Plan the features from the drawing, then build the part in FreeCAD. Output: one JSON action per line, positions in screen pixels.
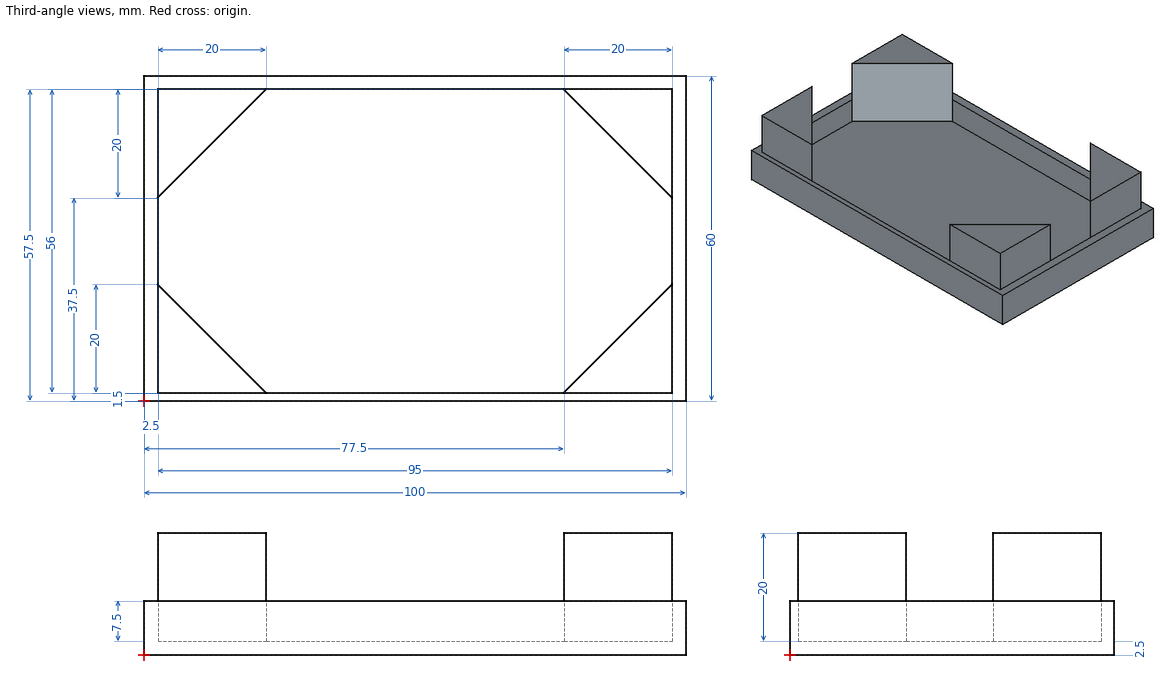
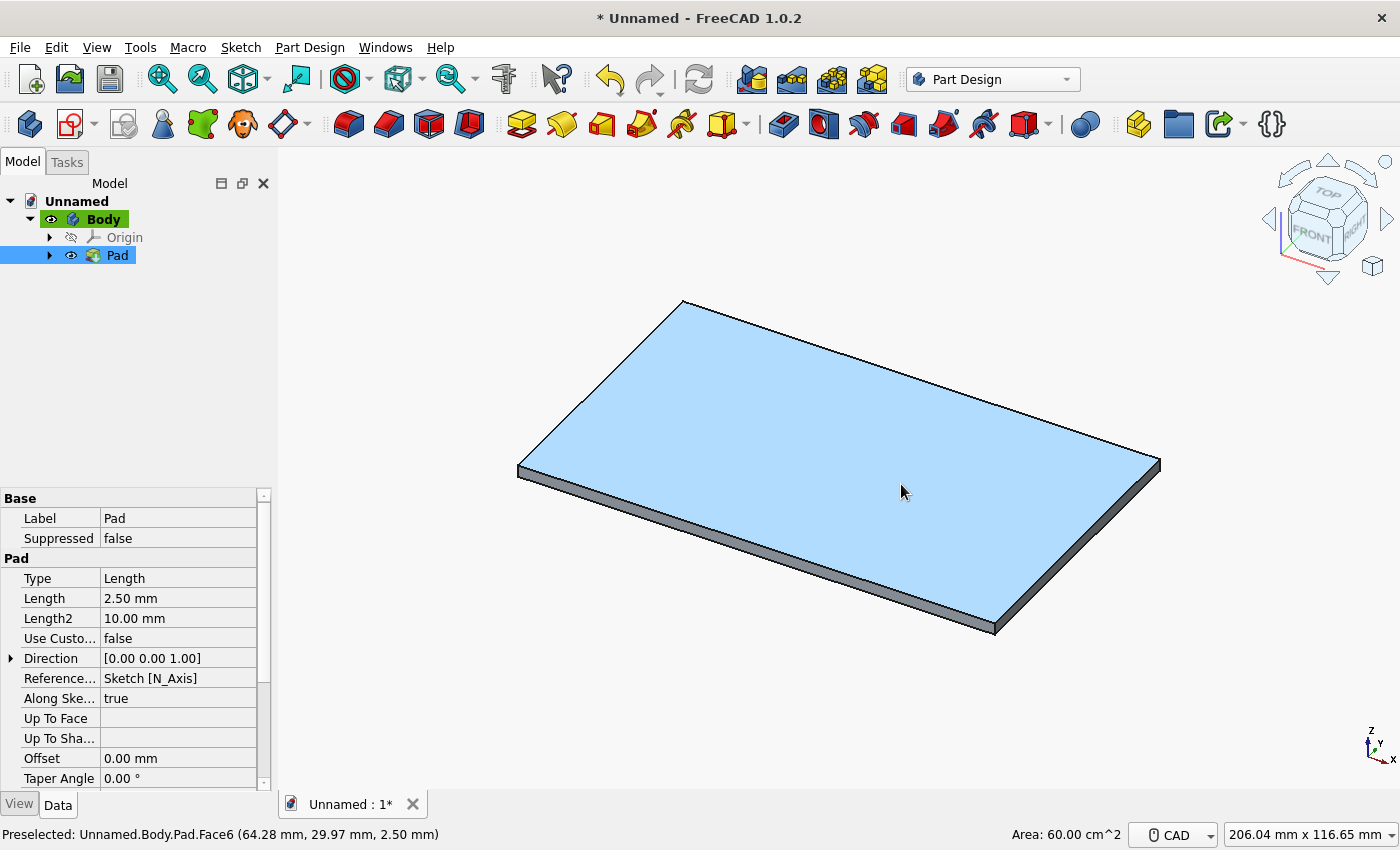
{"action": "left_click", "coordinate": [70, 124]}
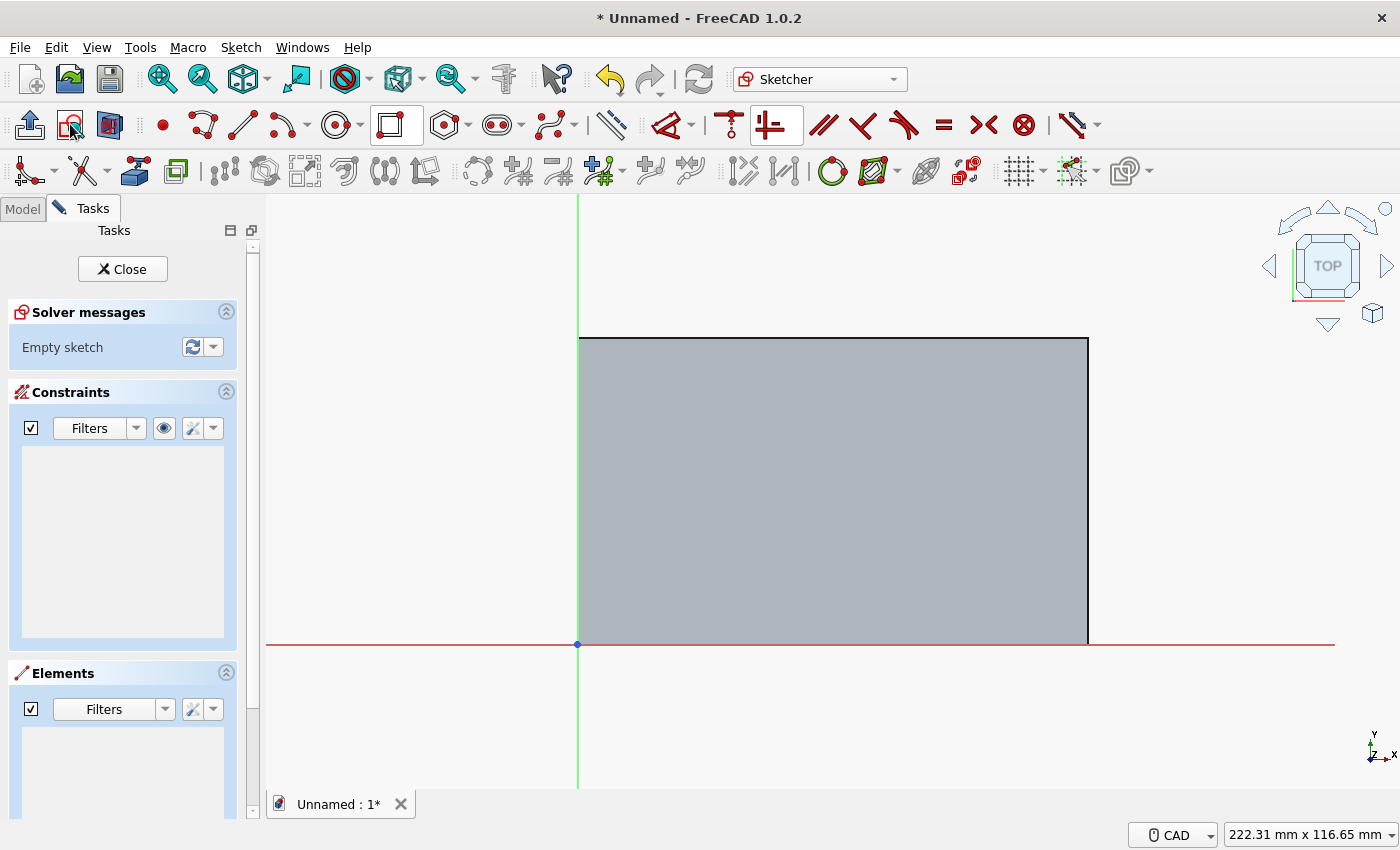
{"action": "left_click", "coordinate": [390, 126]}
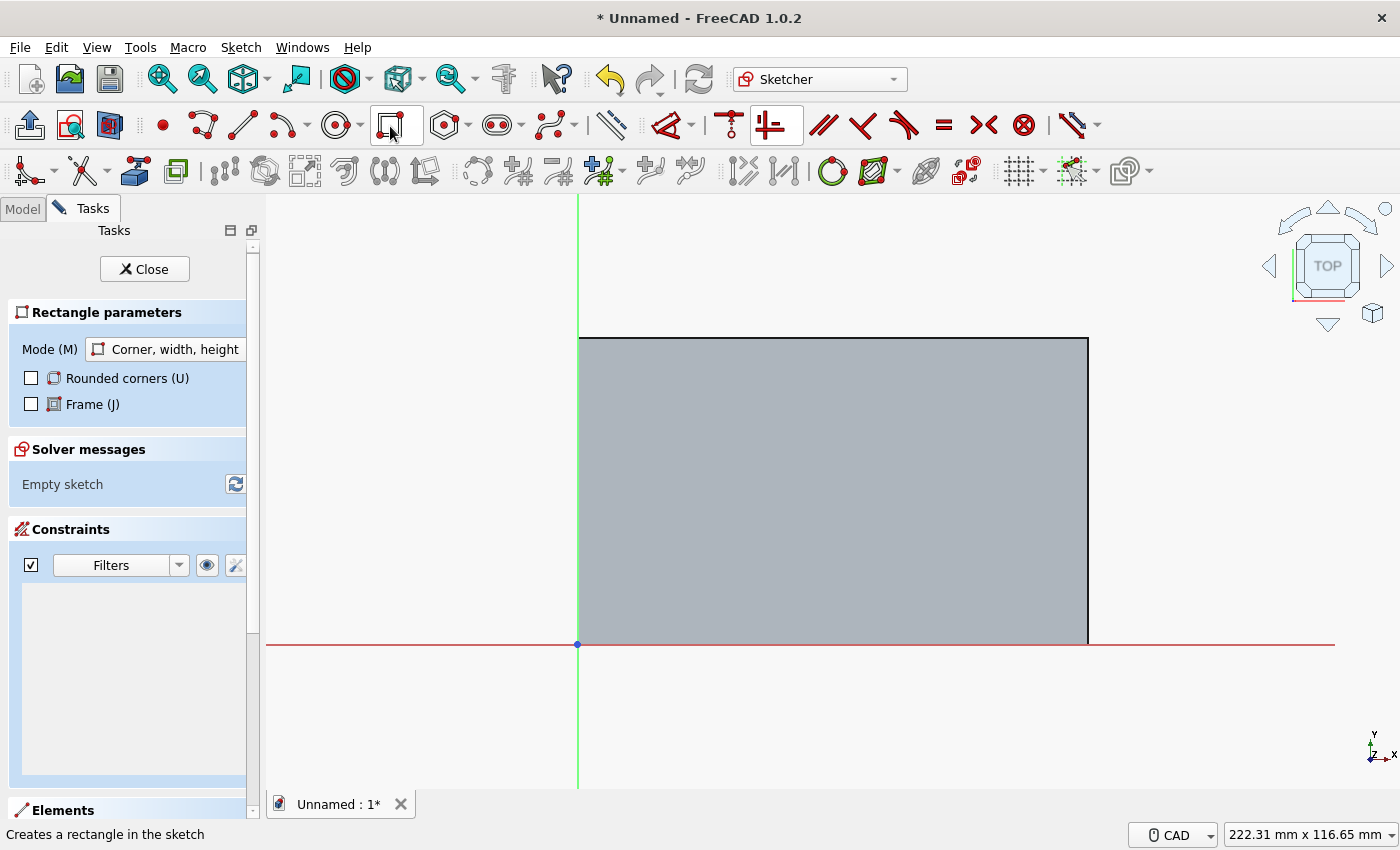
{"action": "left_click", "coordinate": [578, 645]}
{"action": "mouse_move", "coordinate": [1088, 338]}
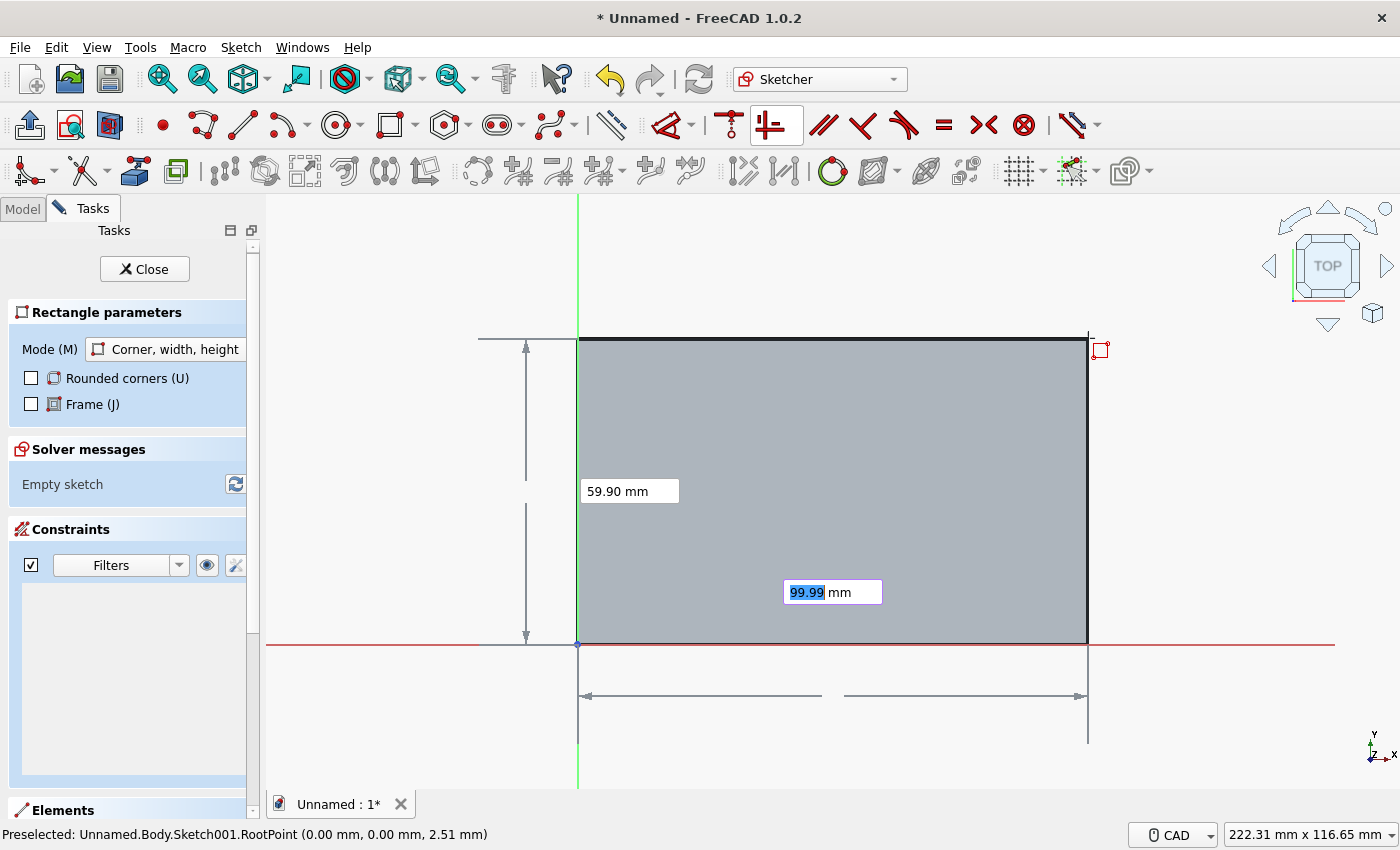
{"action": "type", "text": "100"}
{"action": "key", "text": "Tab"}
{"action": "type", "text": "60"}
{"action": "key", "text": "Return"}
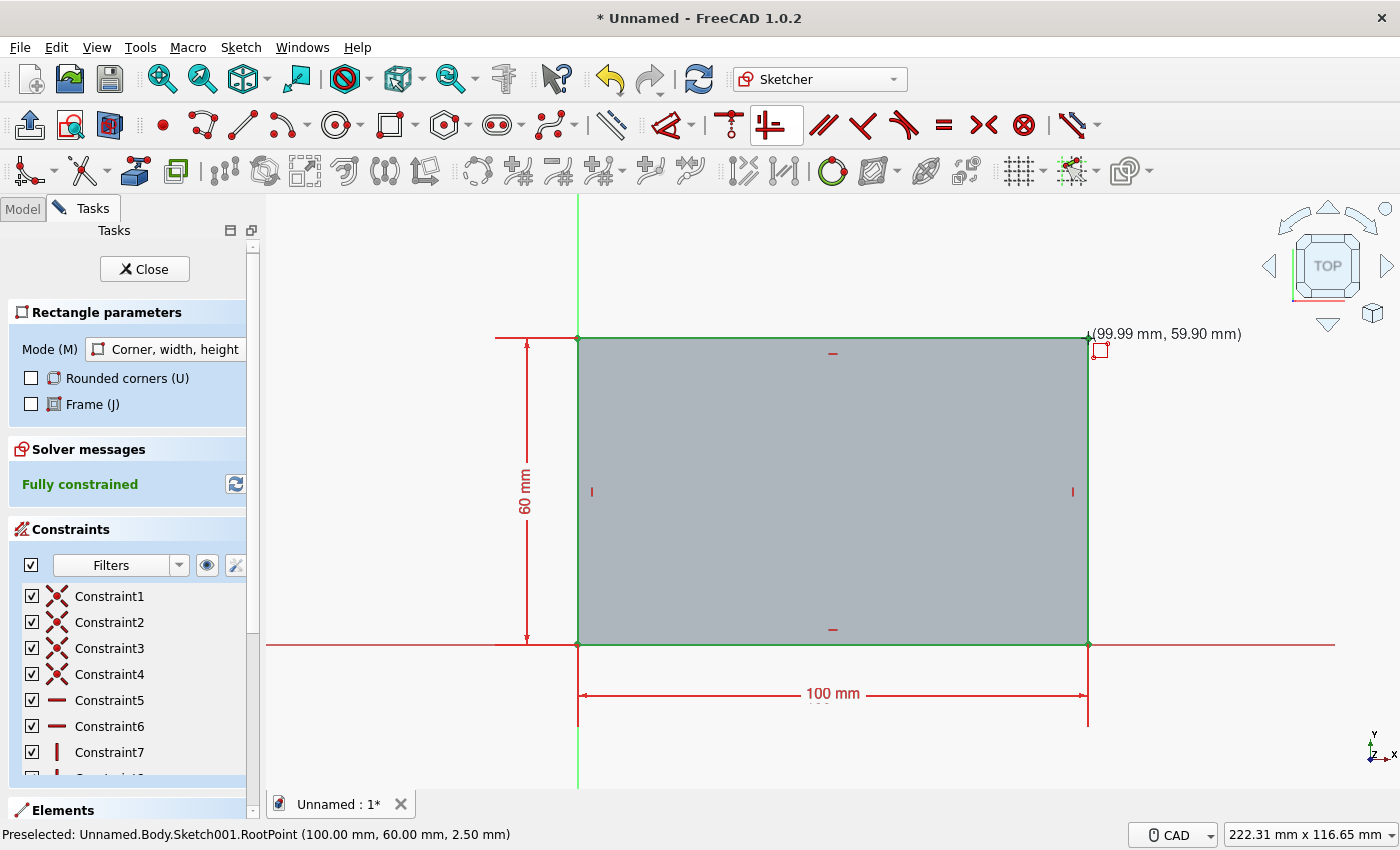
{"action": "scroll", "coordinate": [591, 351], "scroll_direction": "up", "scroll_amount": 2}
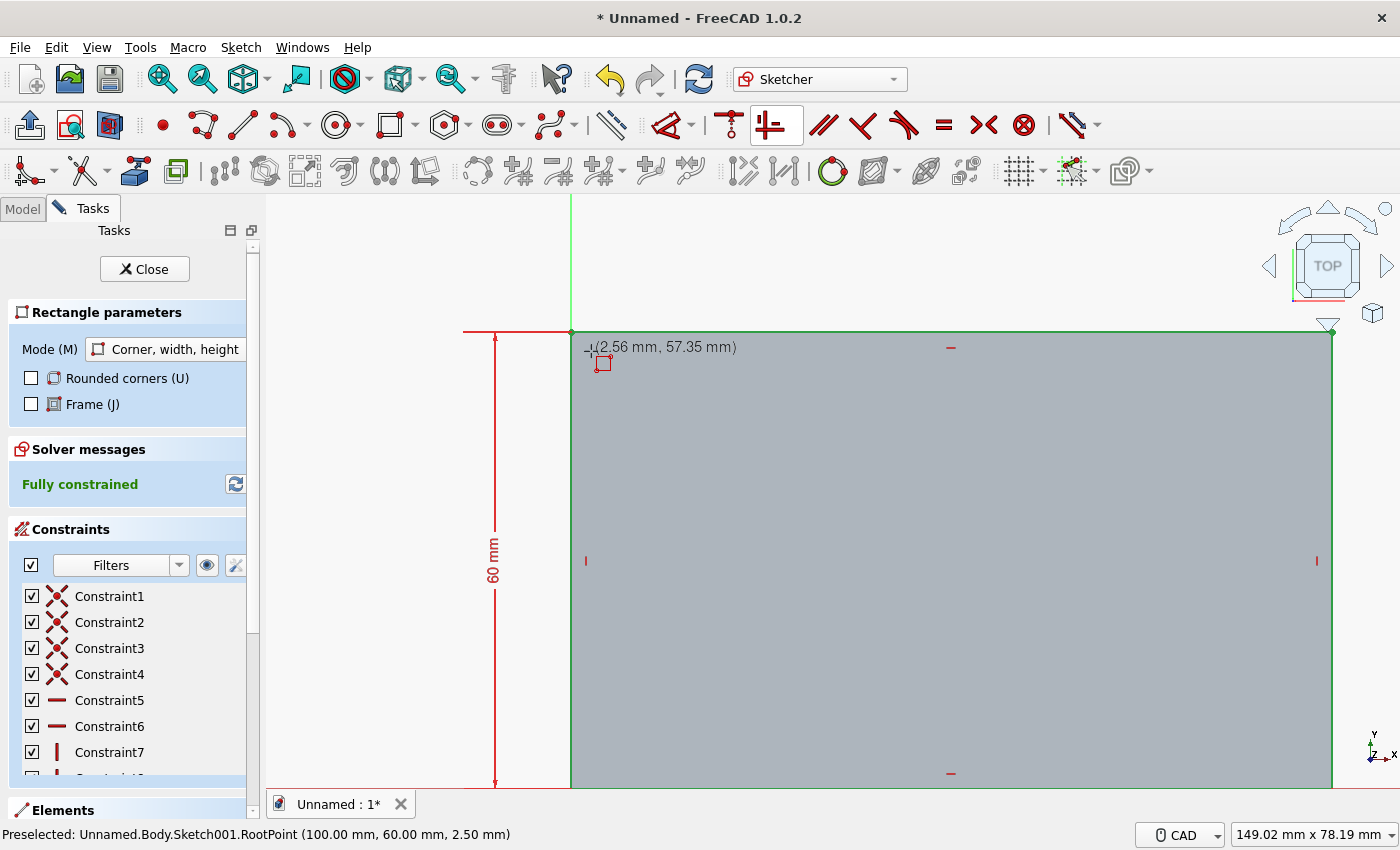
{"action": "left_click", "coordinate": [590, 351]}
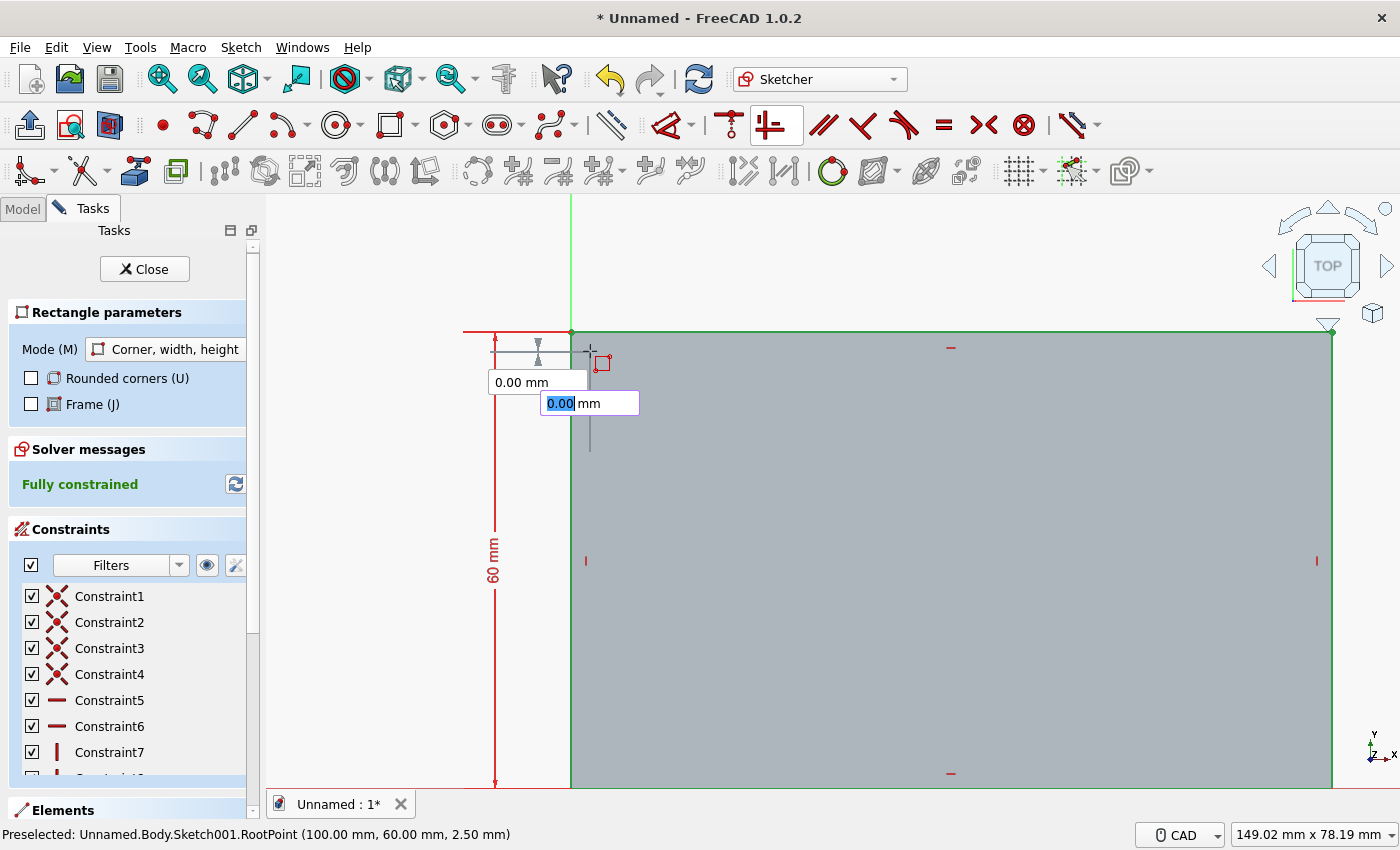
{"action": "scroll", "coordinate": [294, 222], "scroll_direction": "down", "scroll_amount": 1}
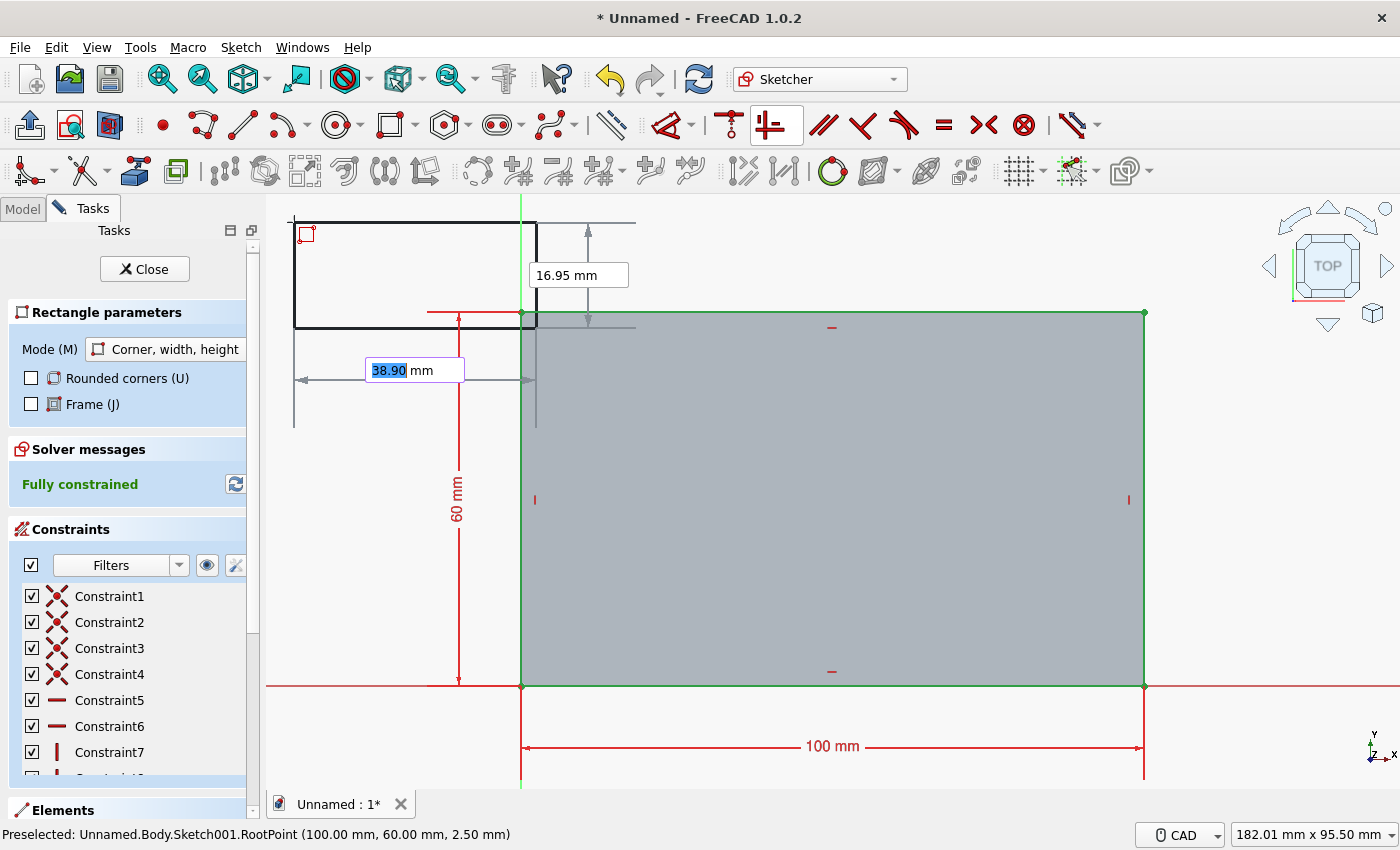
{"action": "scroll", "coordinate": [1129, 677], "scroll_direction": "up", "scroll_amount": 3}